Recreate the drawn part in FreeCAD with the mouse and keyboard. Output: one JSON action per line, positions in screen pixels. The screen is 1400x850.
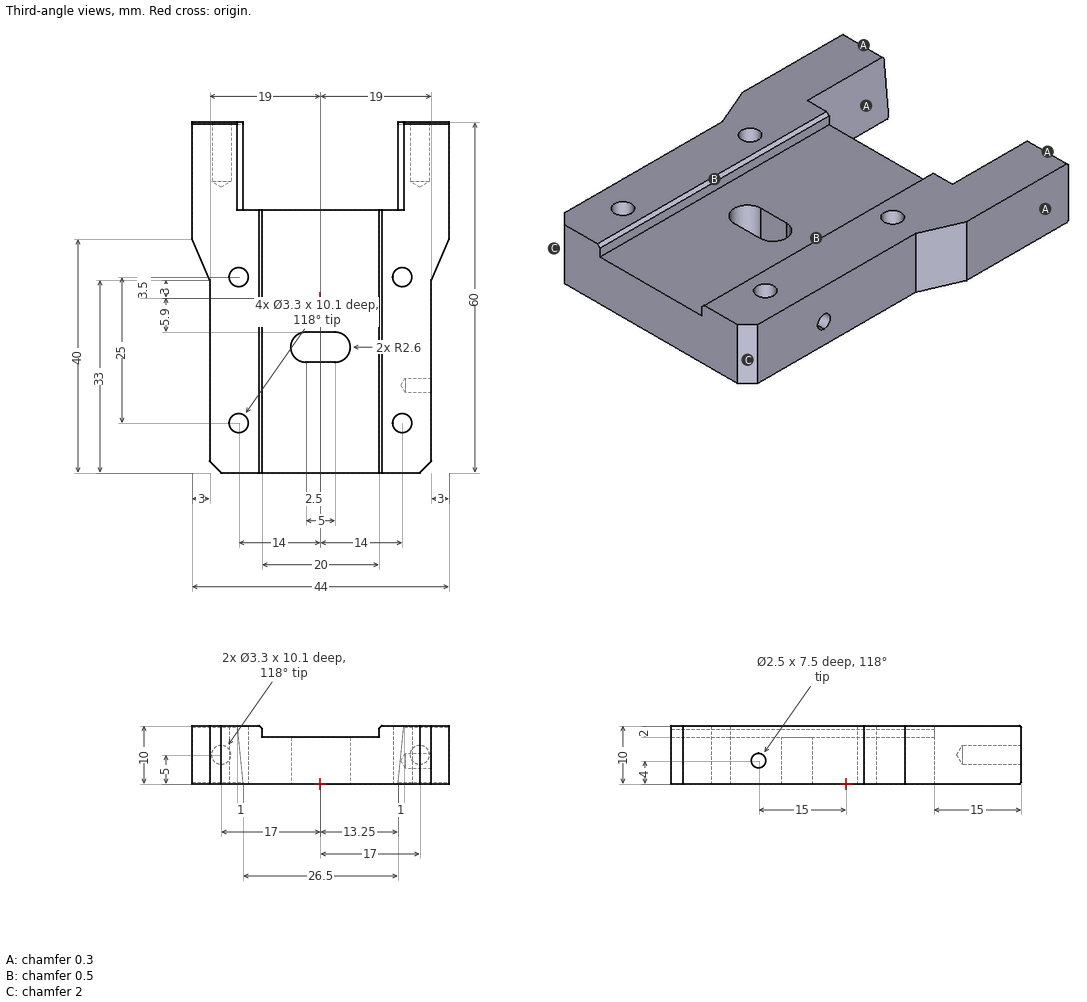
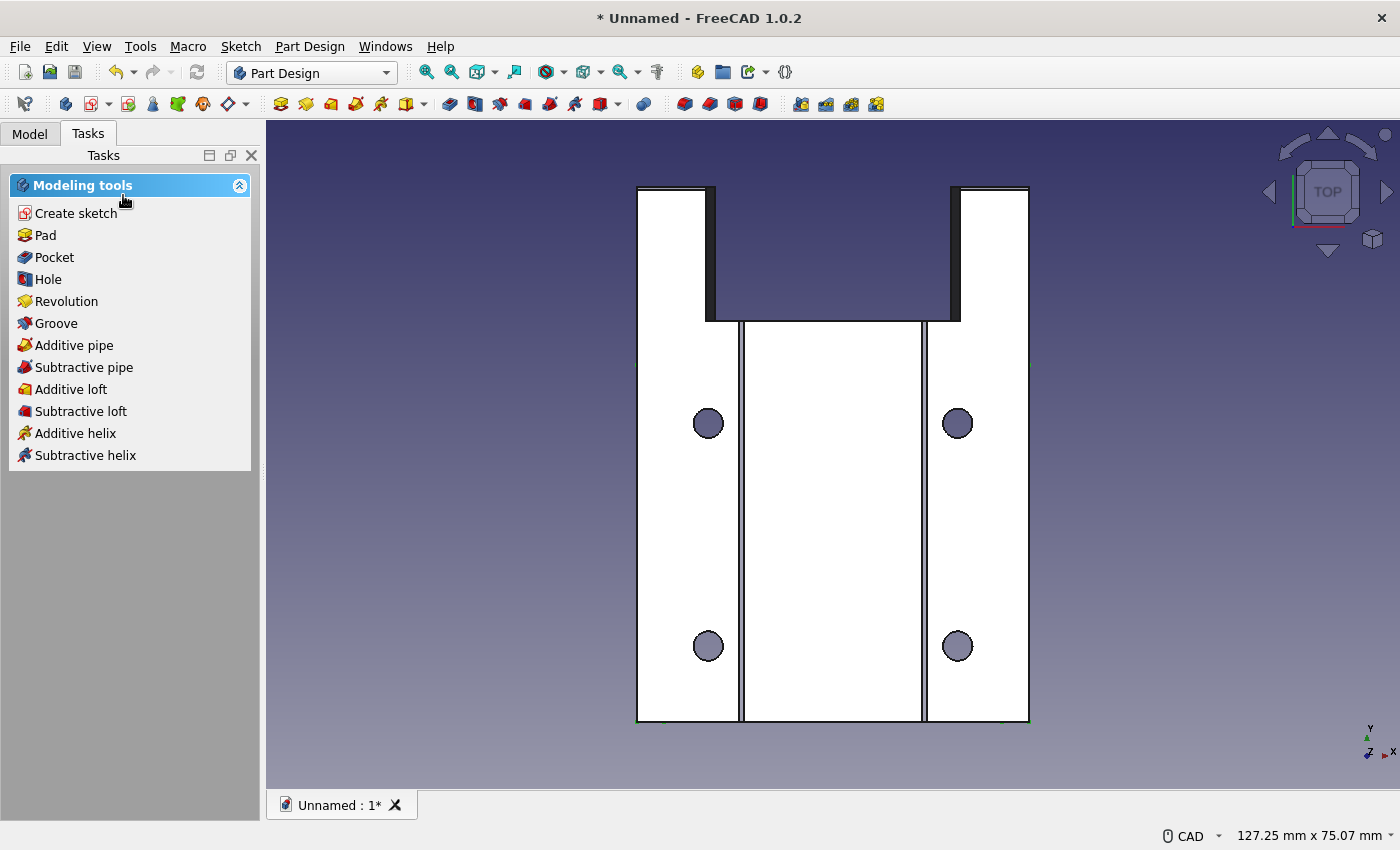
{"action": "left_click", "coordinate": [450, 104]}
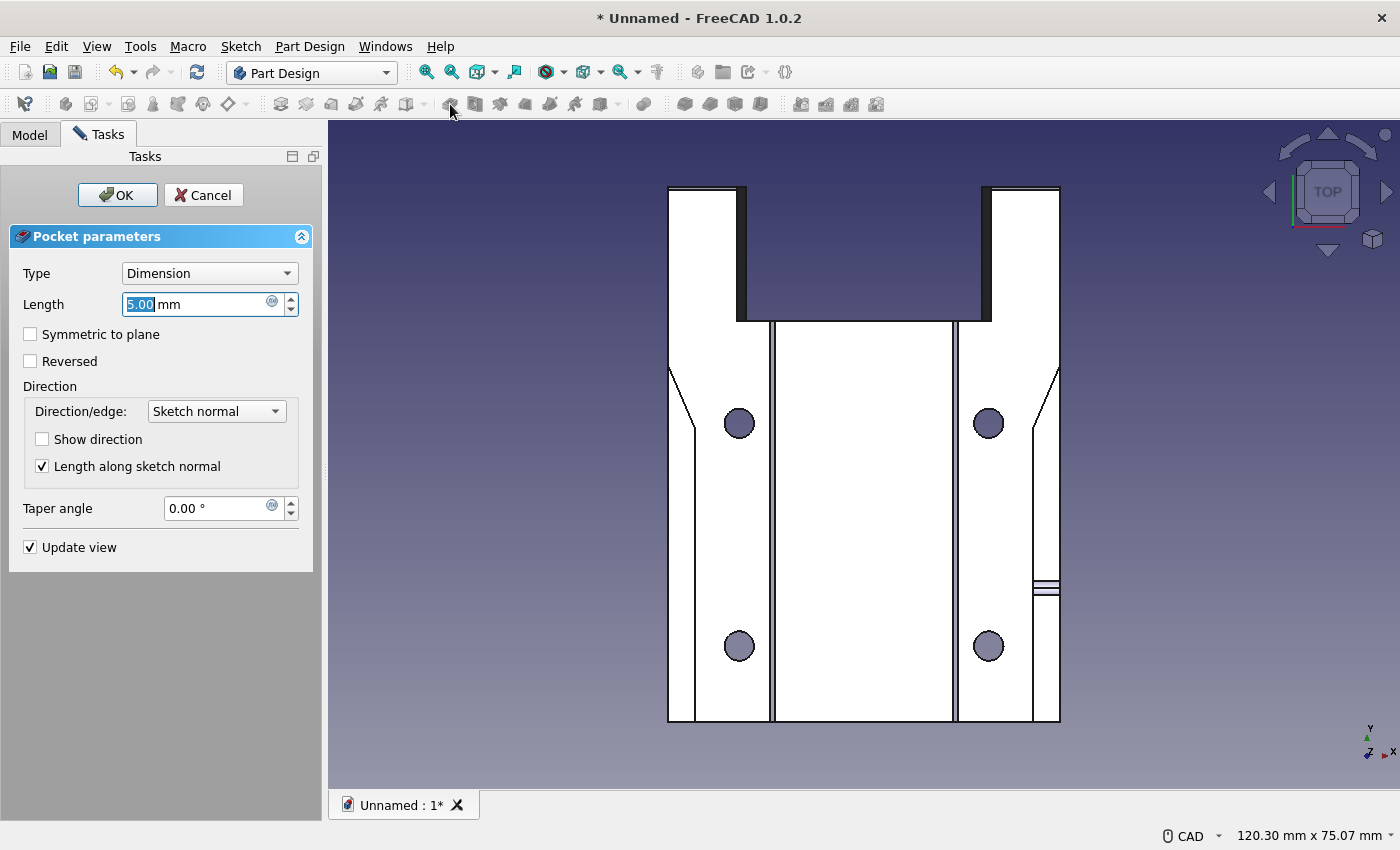
{"action": "left_click", "coordinate": [210, 274]}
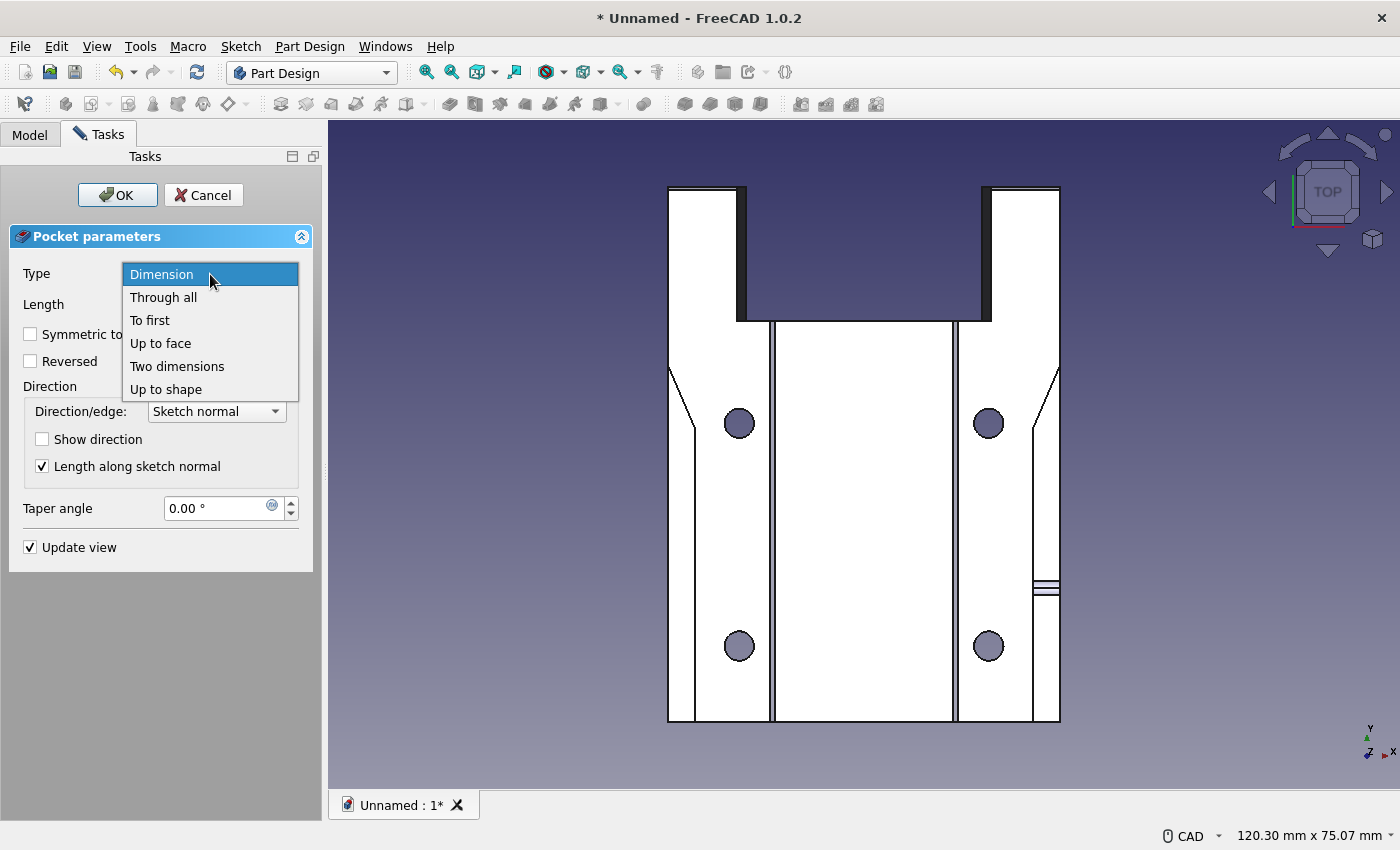
{"action": "left_click", "coordinate": [208, 298]}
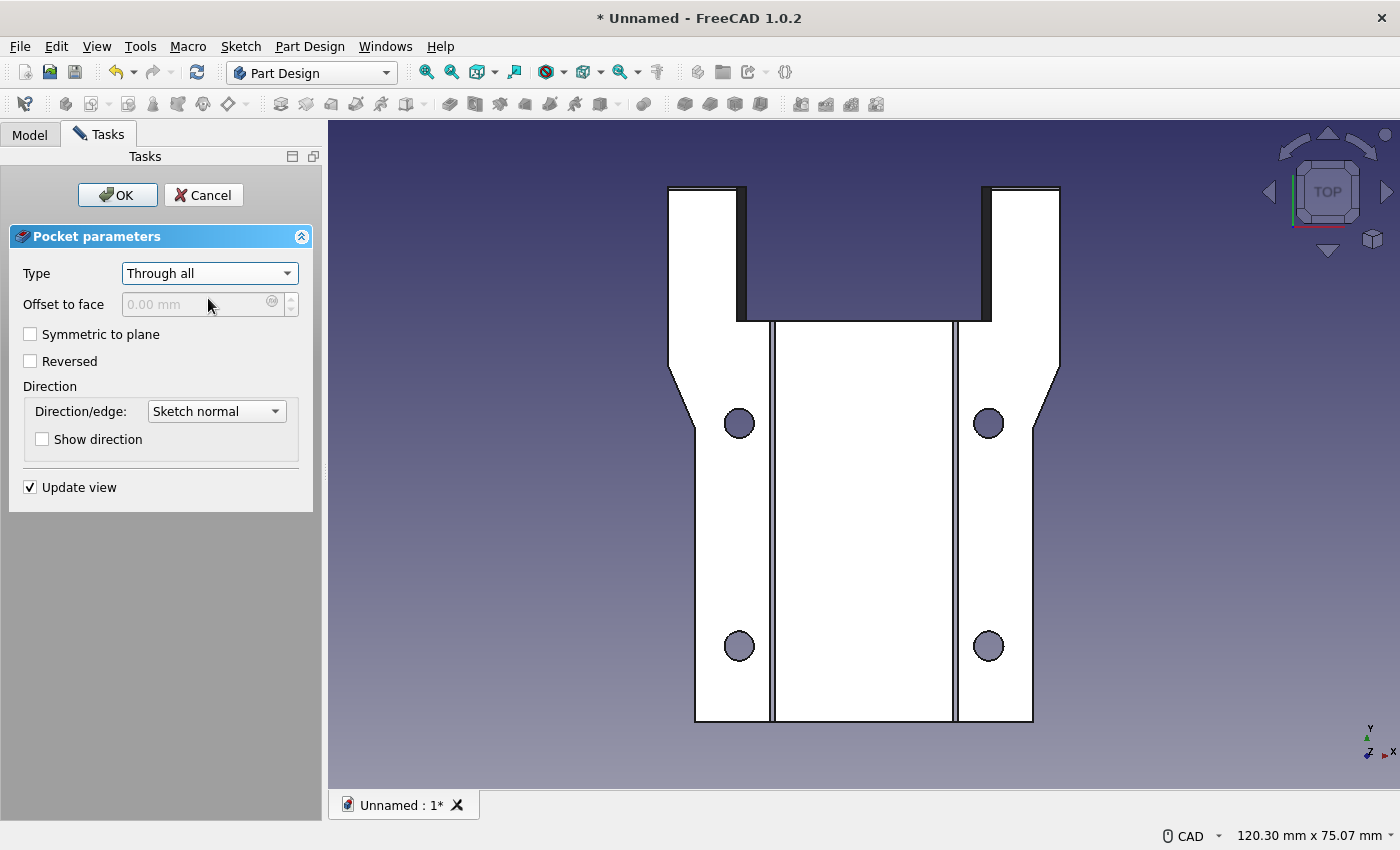
{"action": "left_click", "coordinate": [118, 195]}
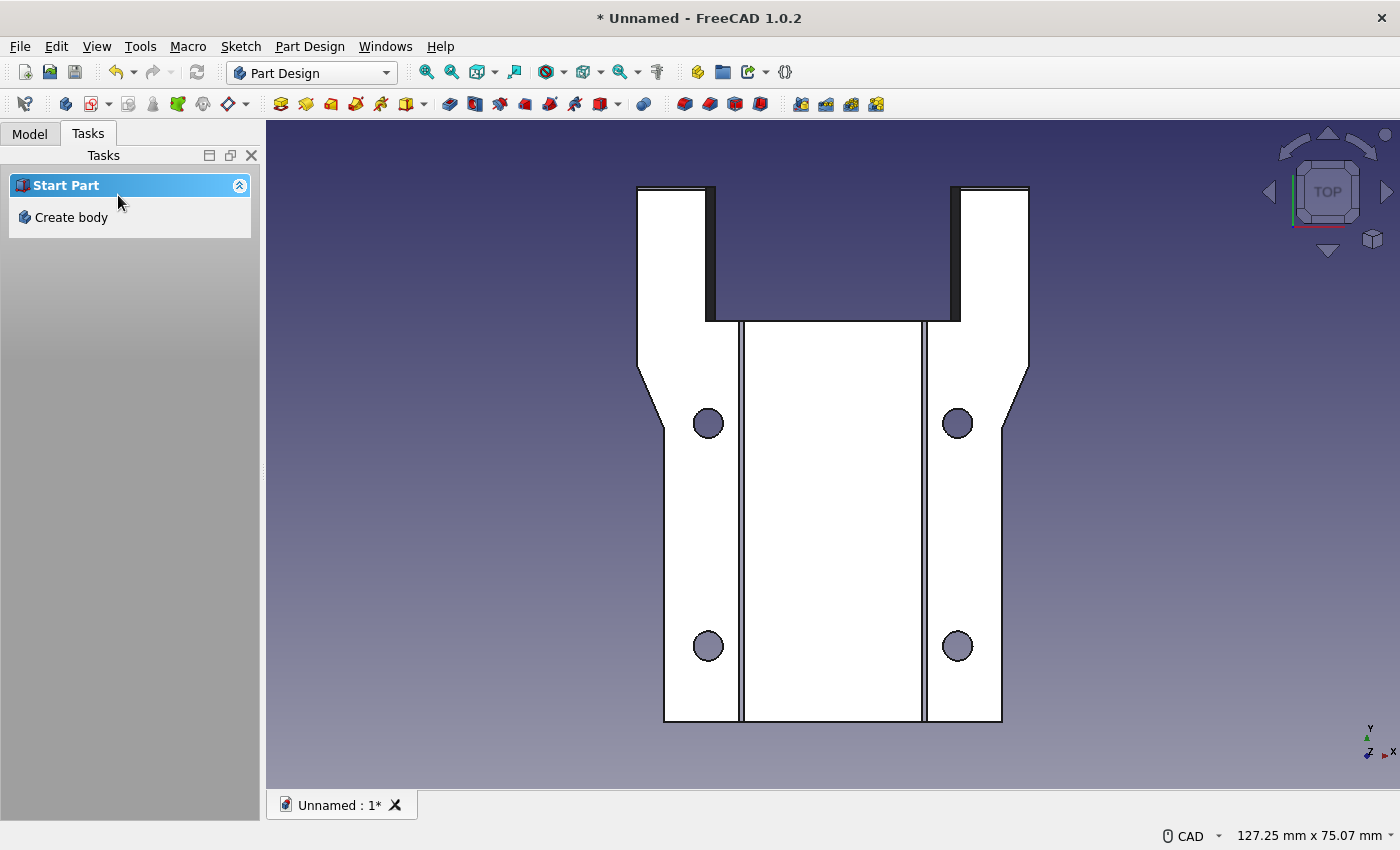
{"action": "key", "text": "0"}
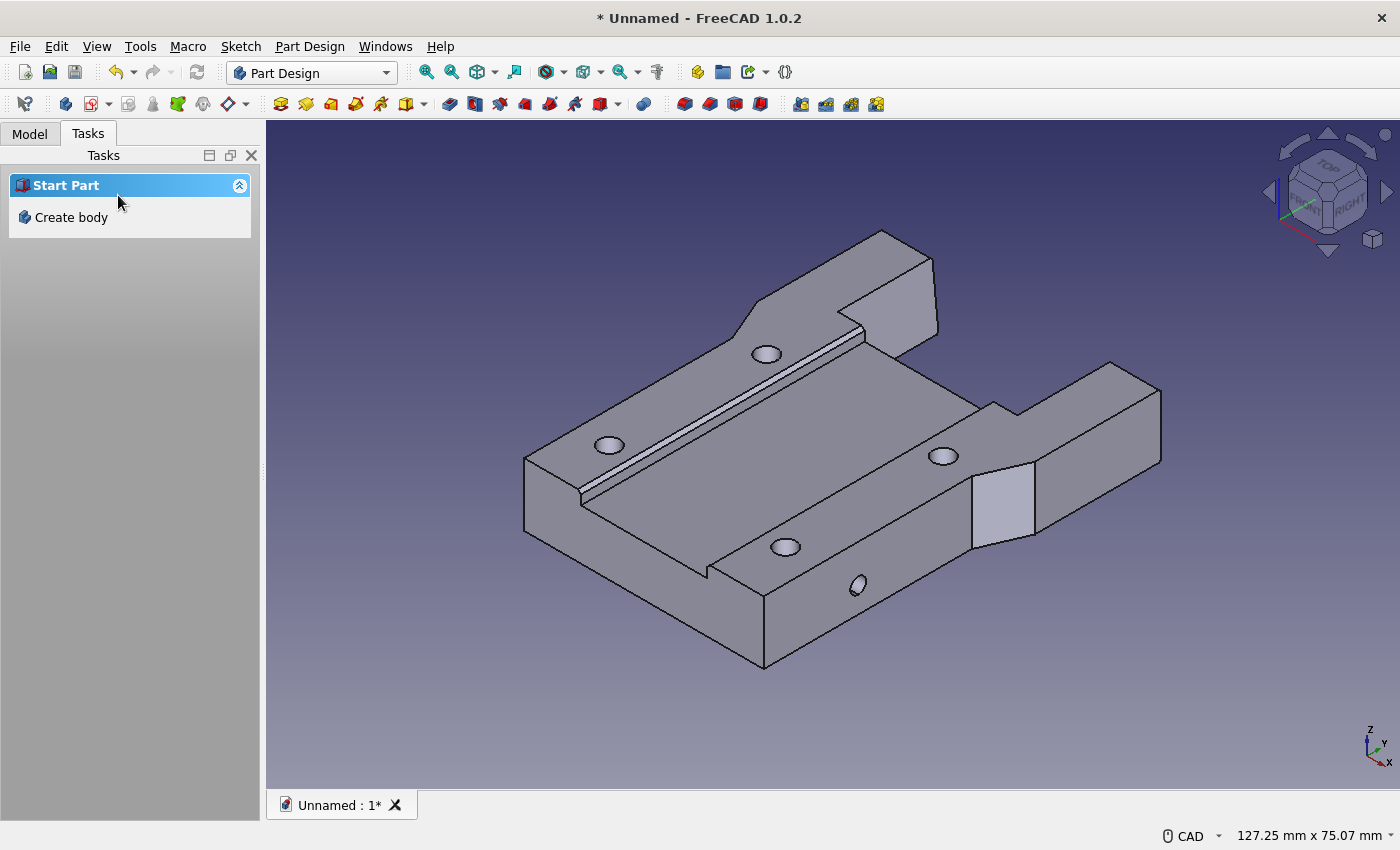
{"action": "left_click", "coordinate": [764, 632]}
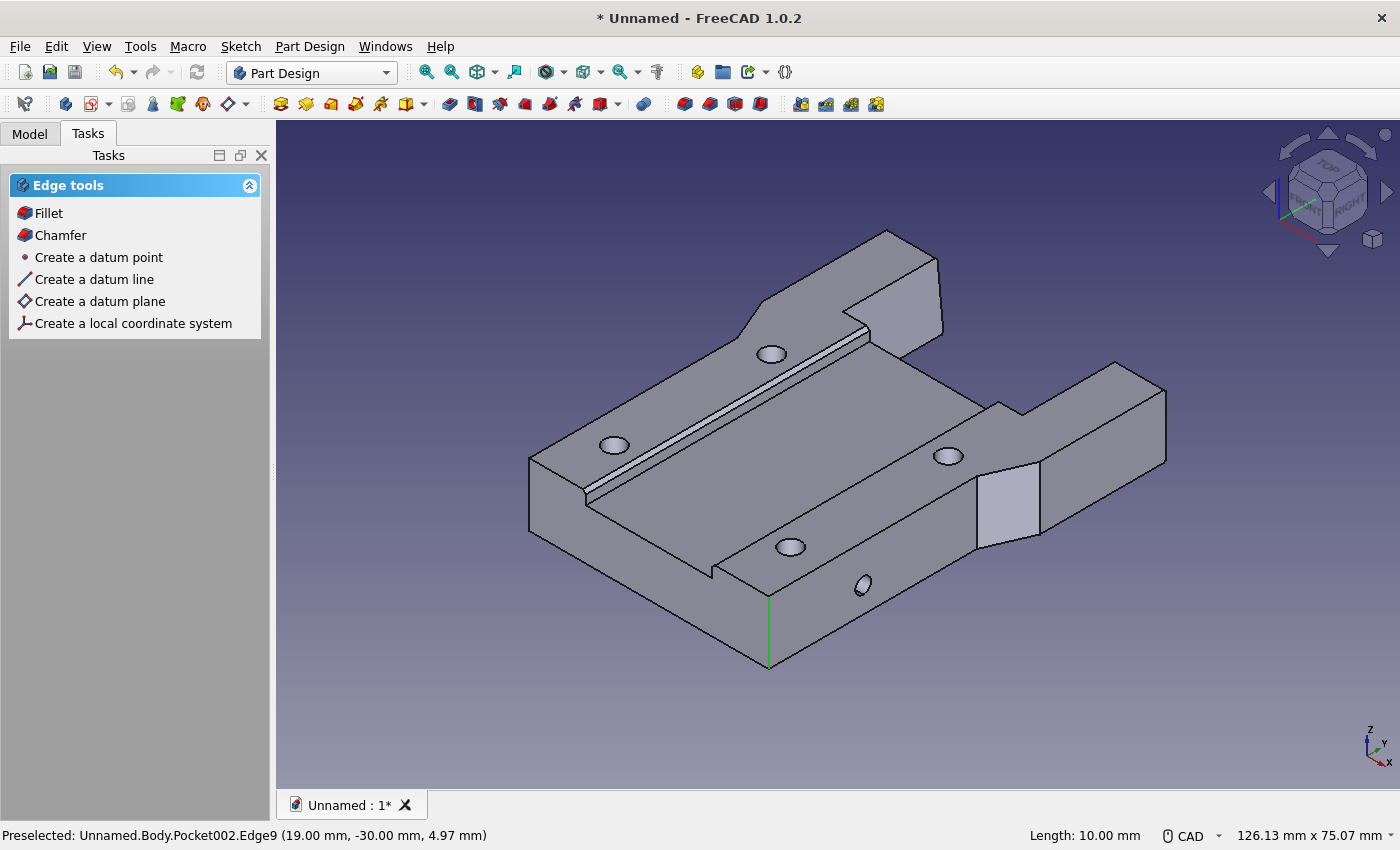
{"action": "key", "text": "2"}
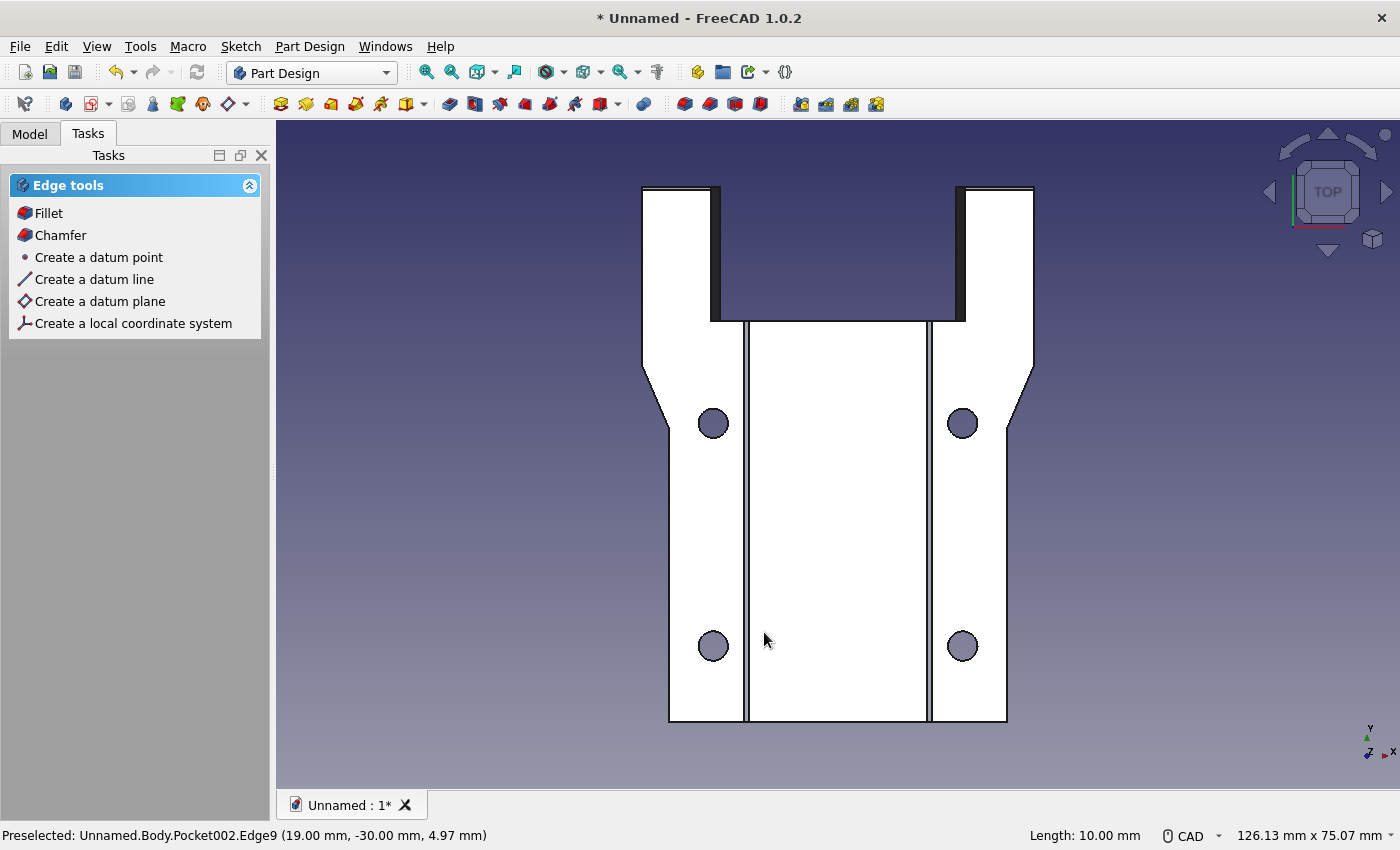
{"action": "key", "text": "1"}